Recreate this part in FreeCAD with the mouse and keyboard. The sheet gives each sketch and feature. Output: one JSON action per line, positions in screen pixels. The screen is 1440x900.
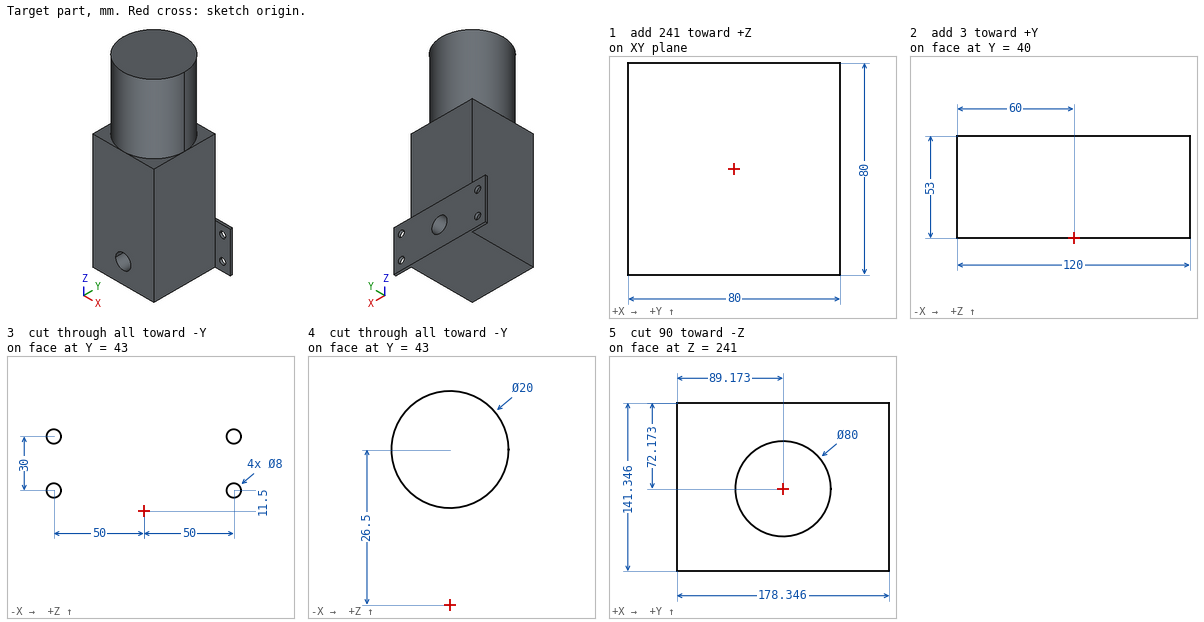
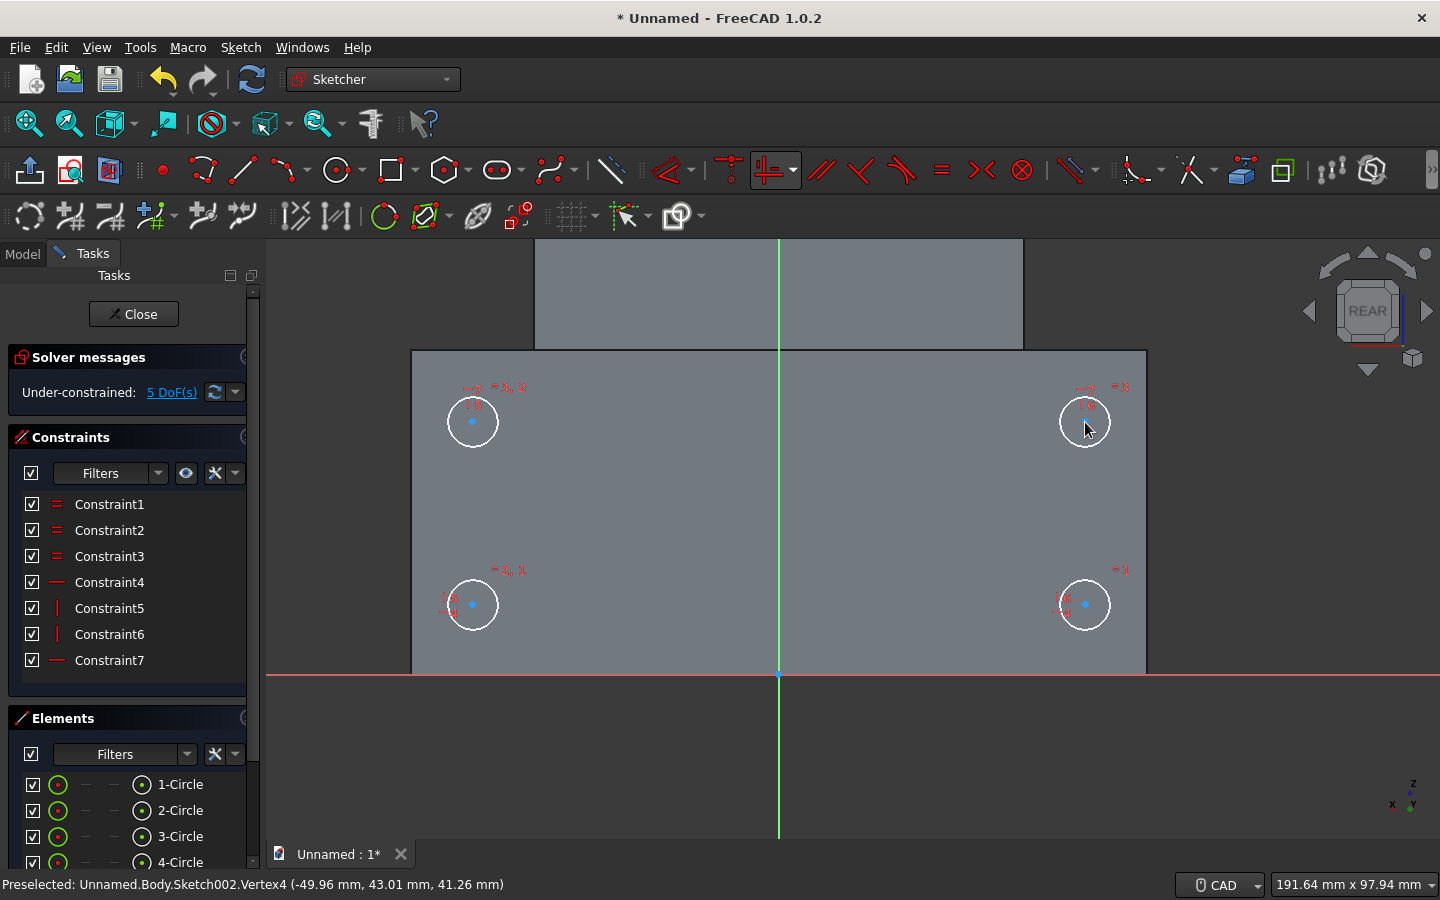
{"action": "key", "text": "d"}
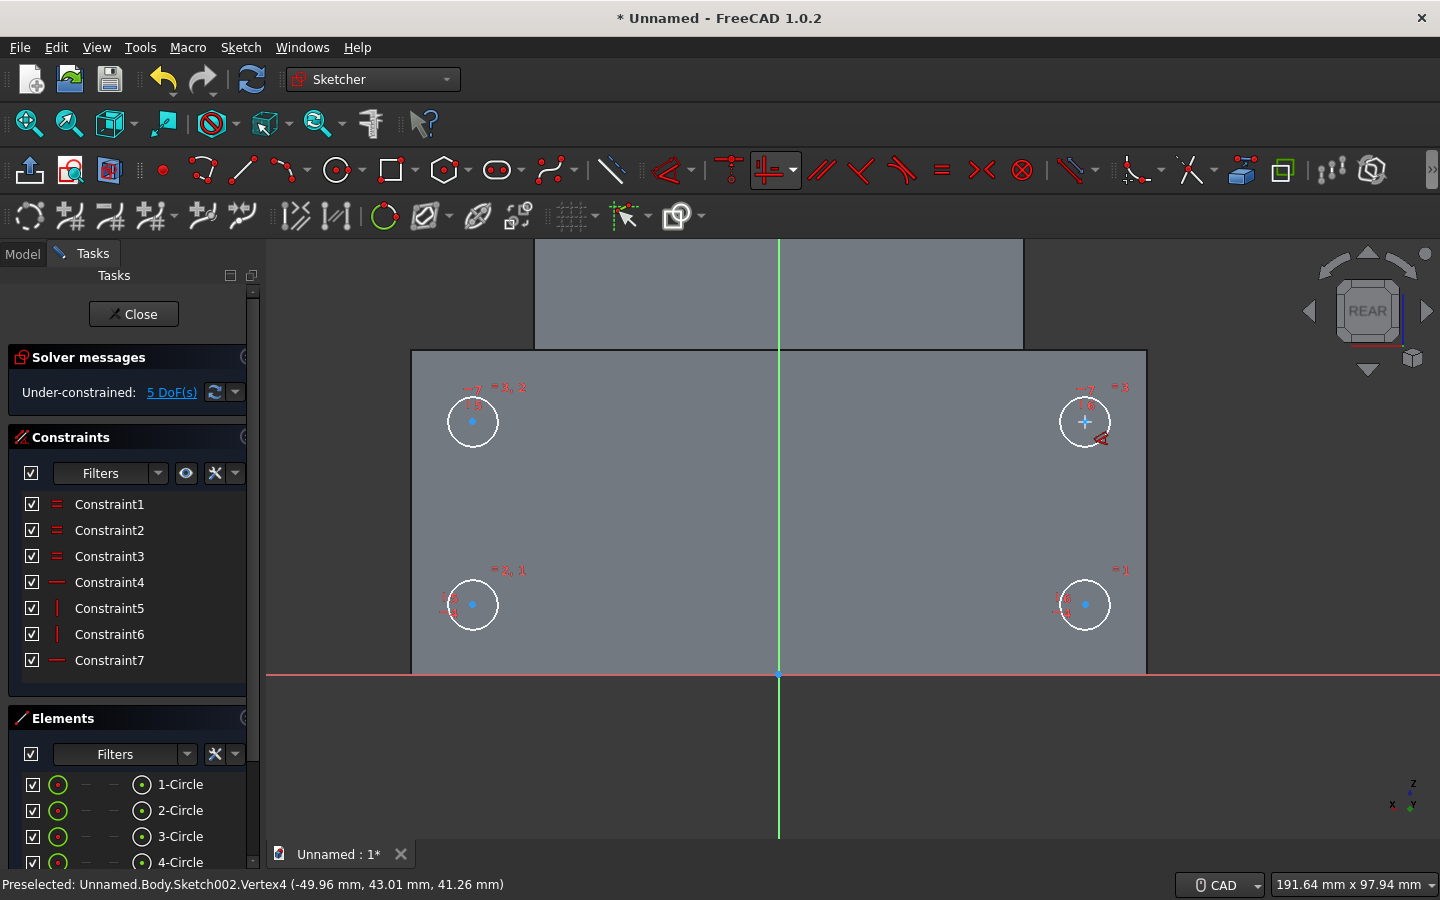
{"action": "left_click", "coordinate": [1102, 587]}
{"action": "left_click", "coordinate": [1124, 564]}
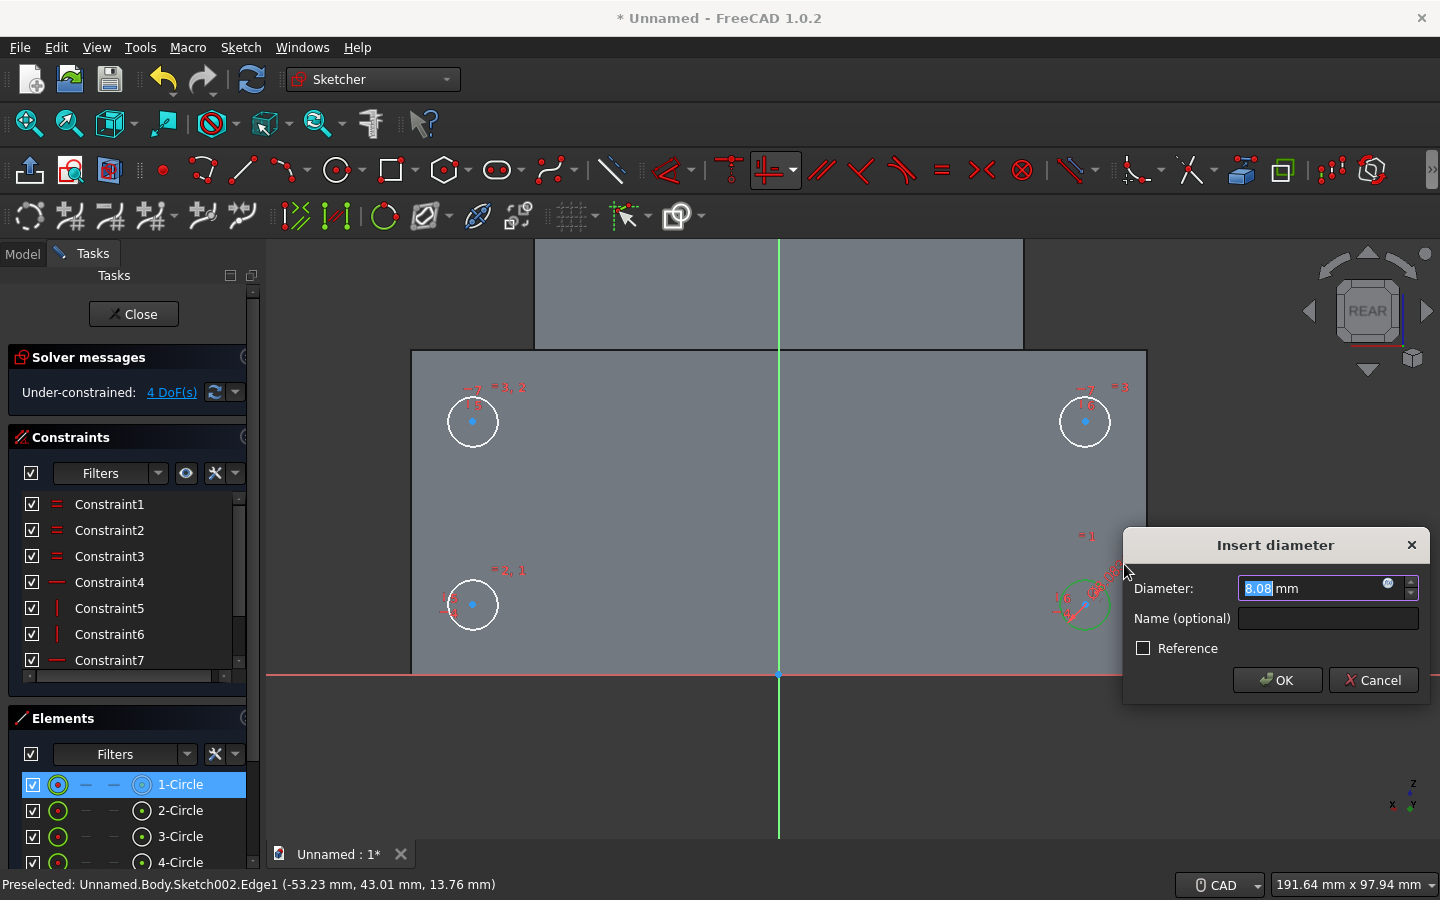
{"action": "type", "text": "8"}
{"action": "key", "text": "Return"}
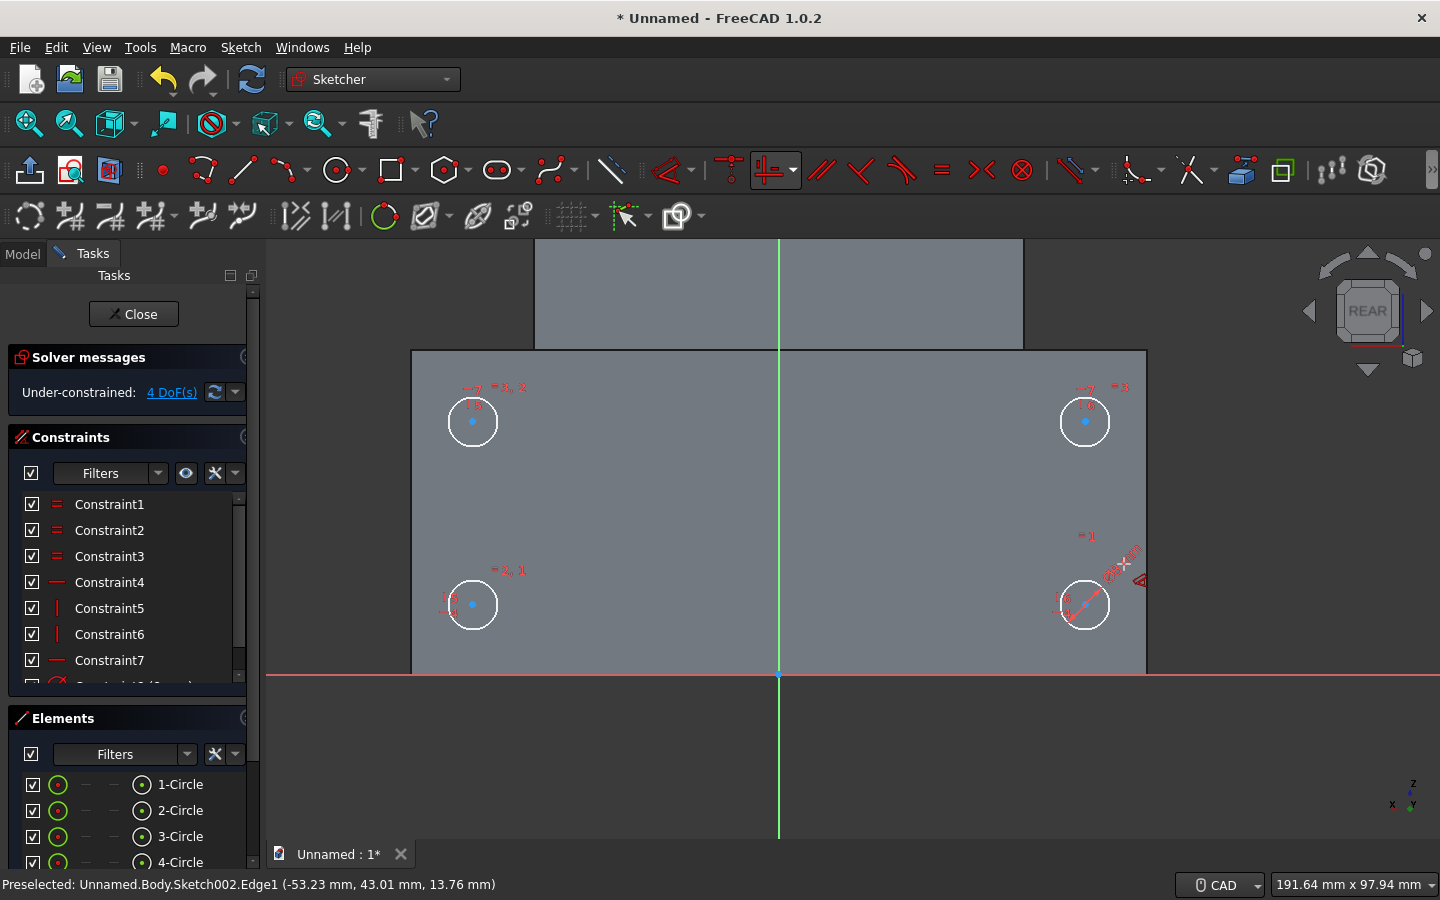
{"action": "left_click", "coordinate": [1085, 605]}
{"action": "left_click", "coordinate": [932, 709]}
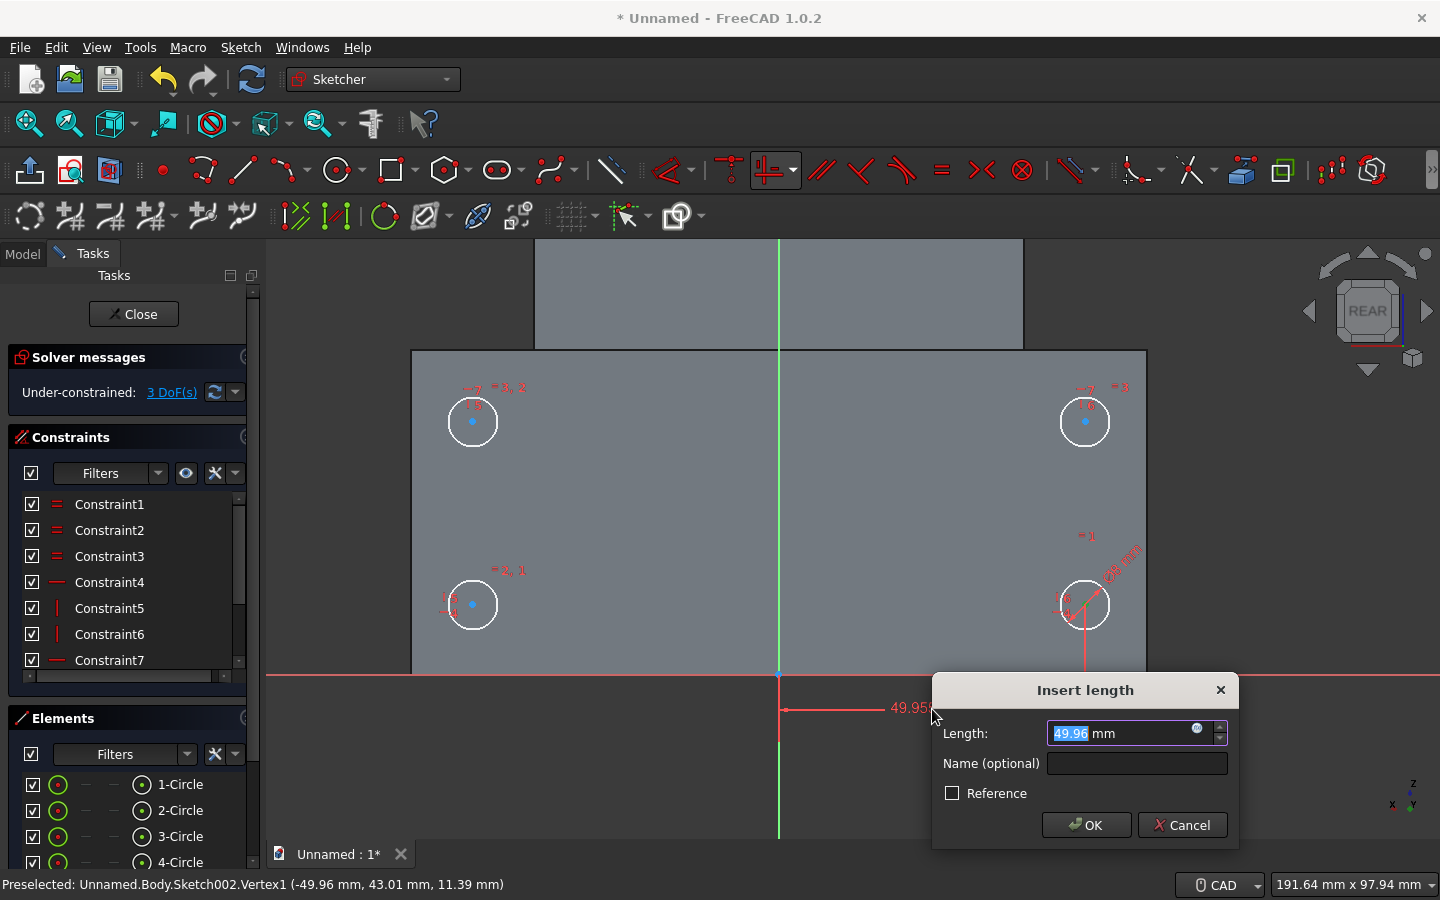
{"action": "type", "text": "50"}
{"action": "key", "text": "Return"}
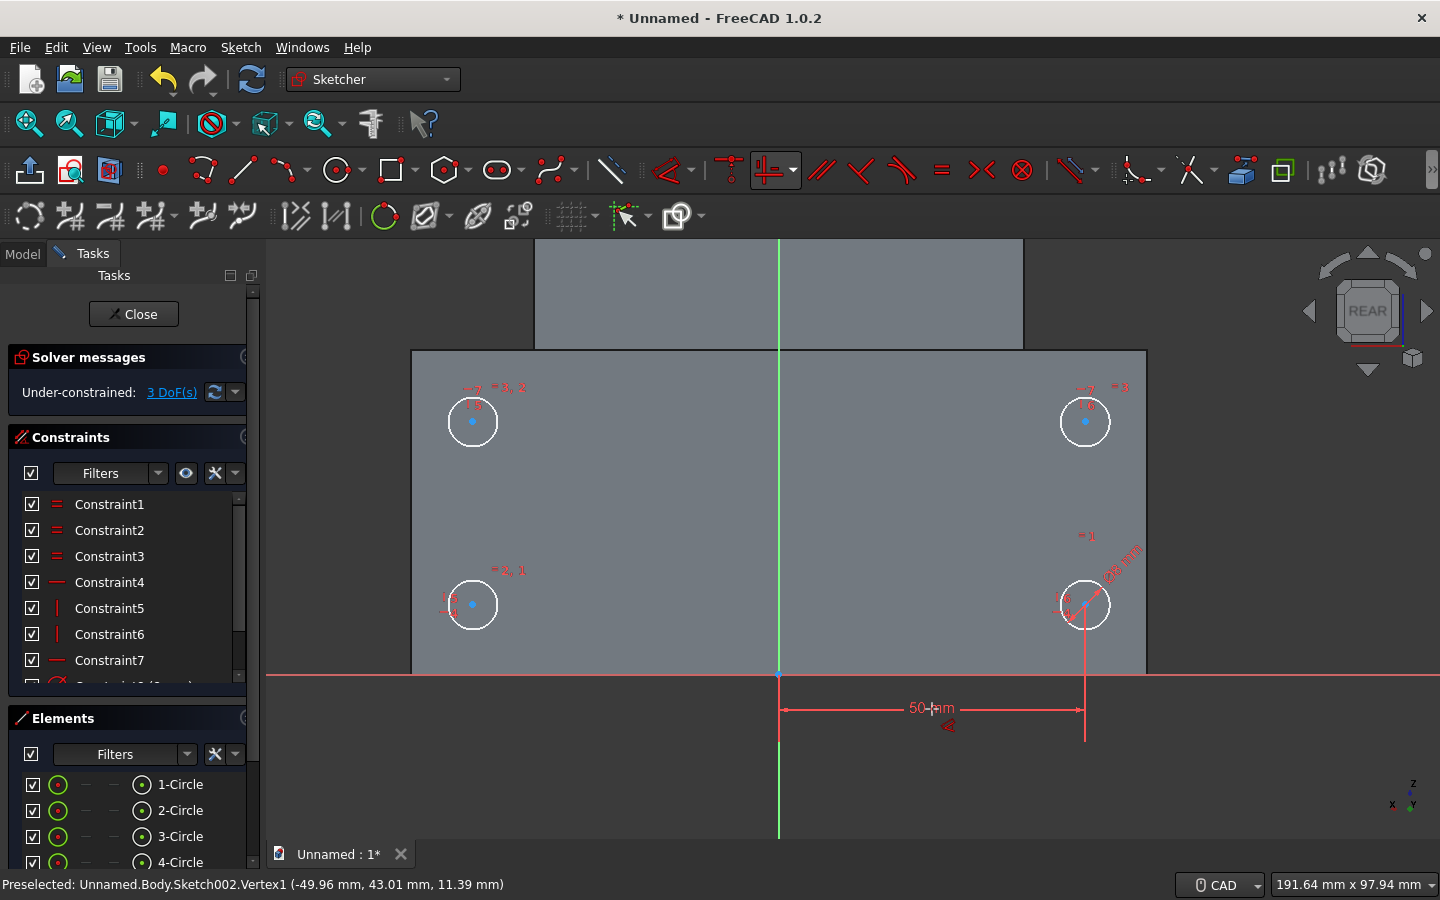
{"action": "left_click", "coordinate": [473, 605]}
{"action": "left_click", "coordinate": [626, 709]}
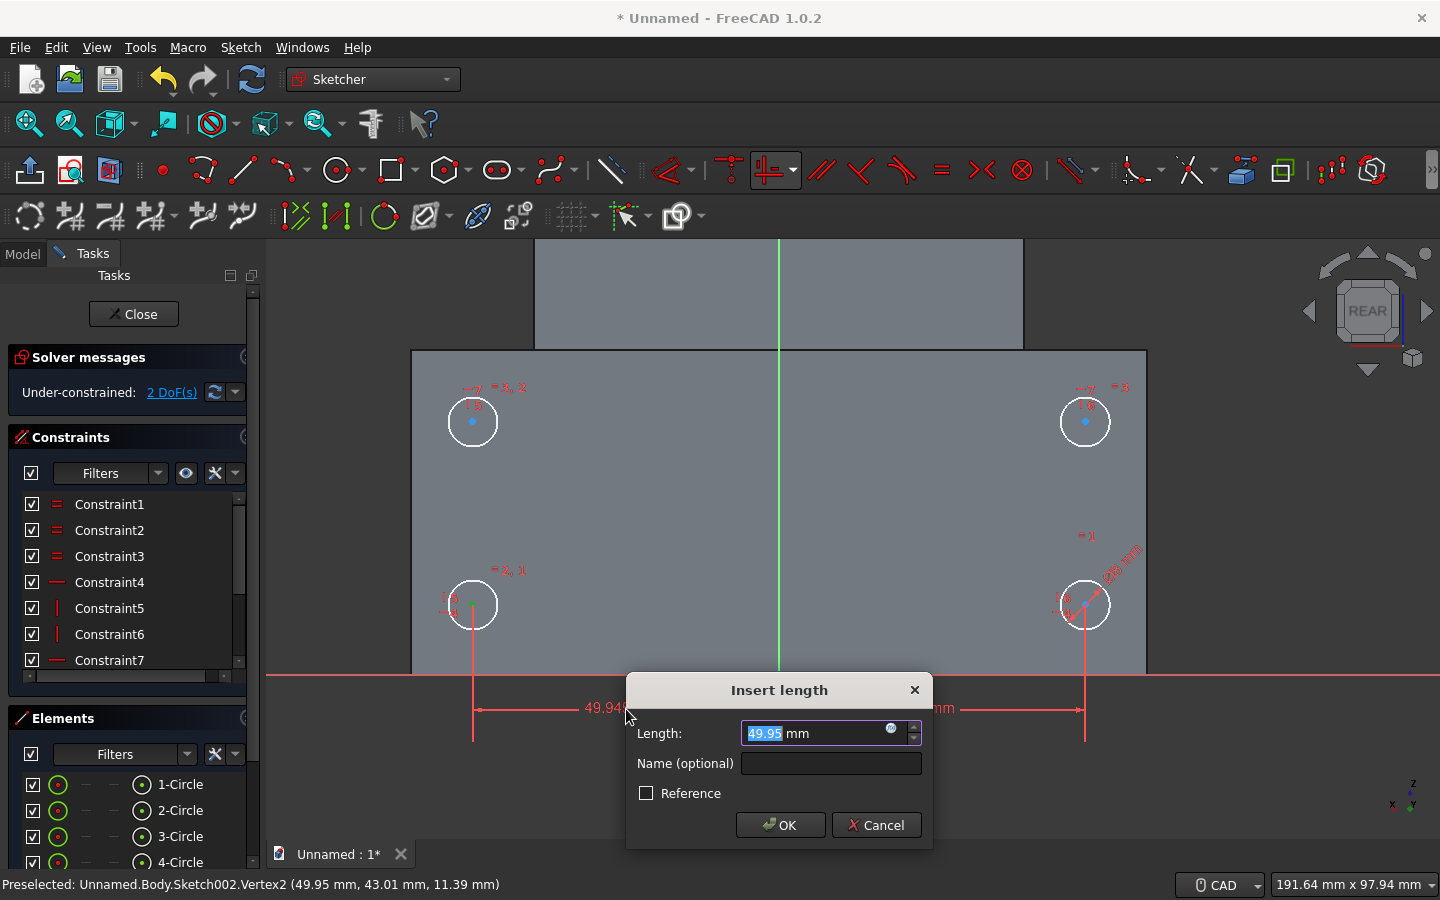
{"action": "type", "text": "50"}
{"action": "key", "text": "Return"}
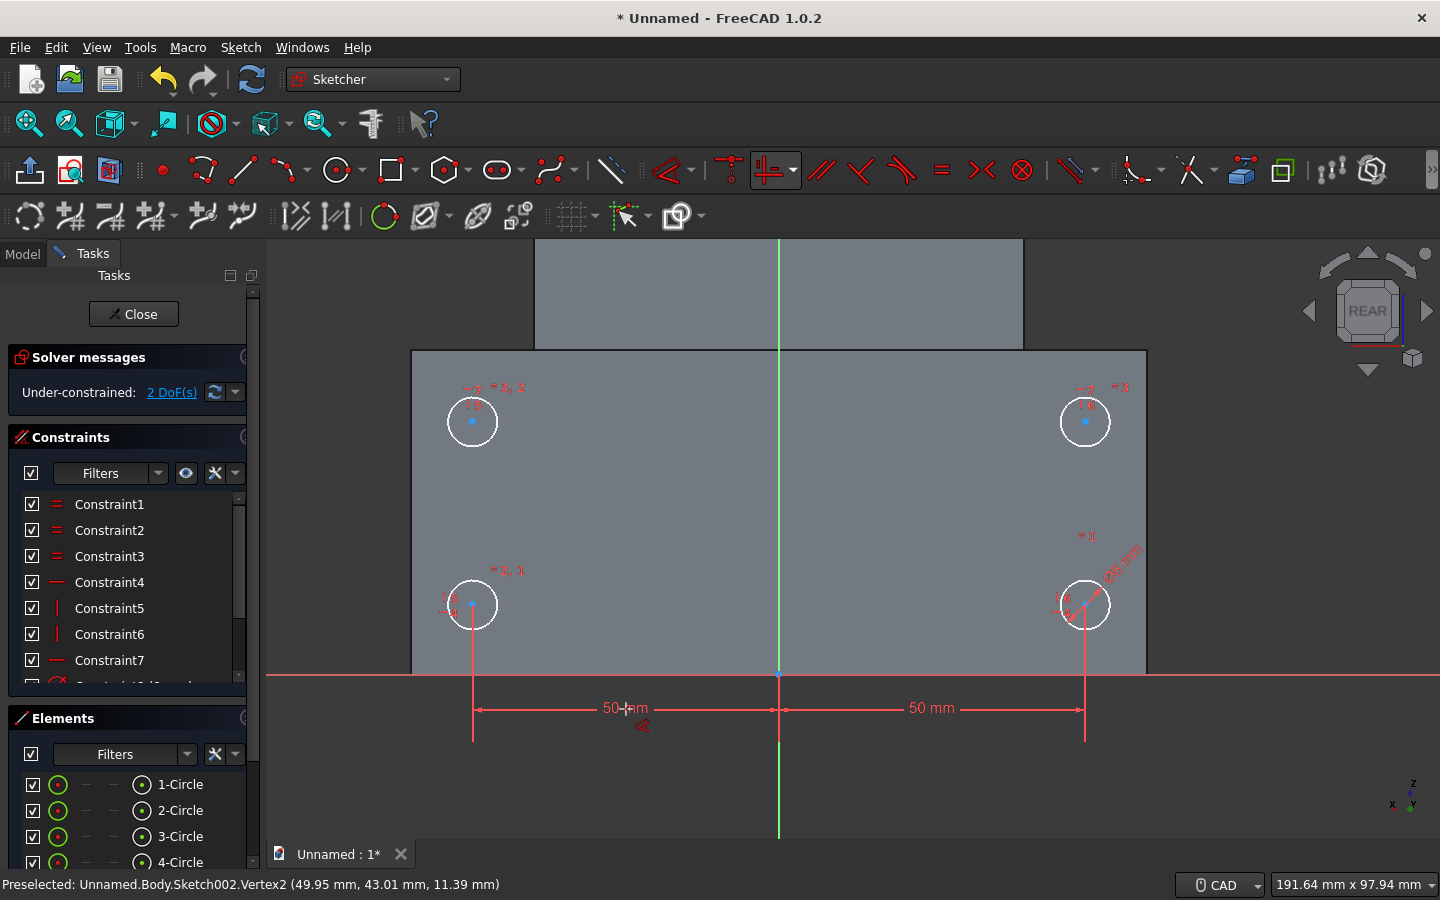
{"action": "left_click", "coordinate": [473, 605]}